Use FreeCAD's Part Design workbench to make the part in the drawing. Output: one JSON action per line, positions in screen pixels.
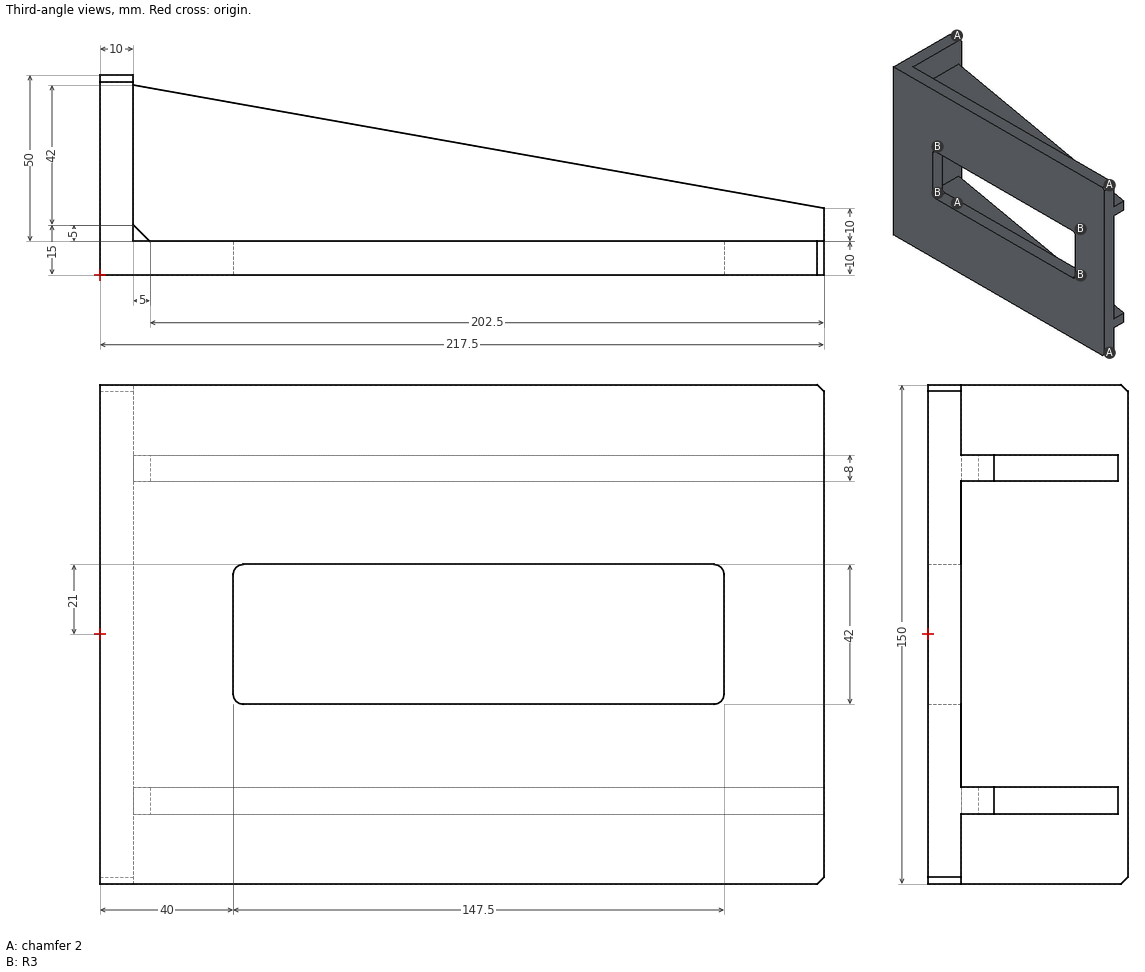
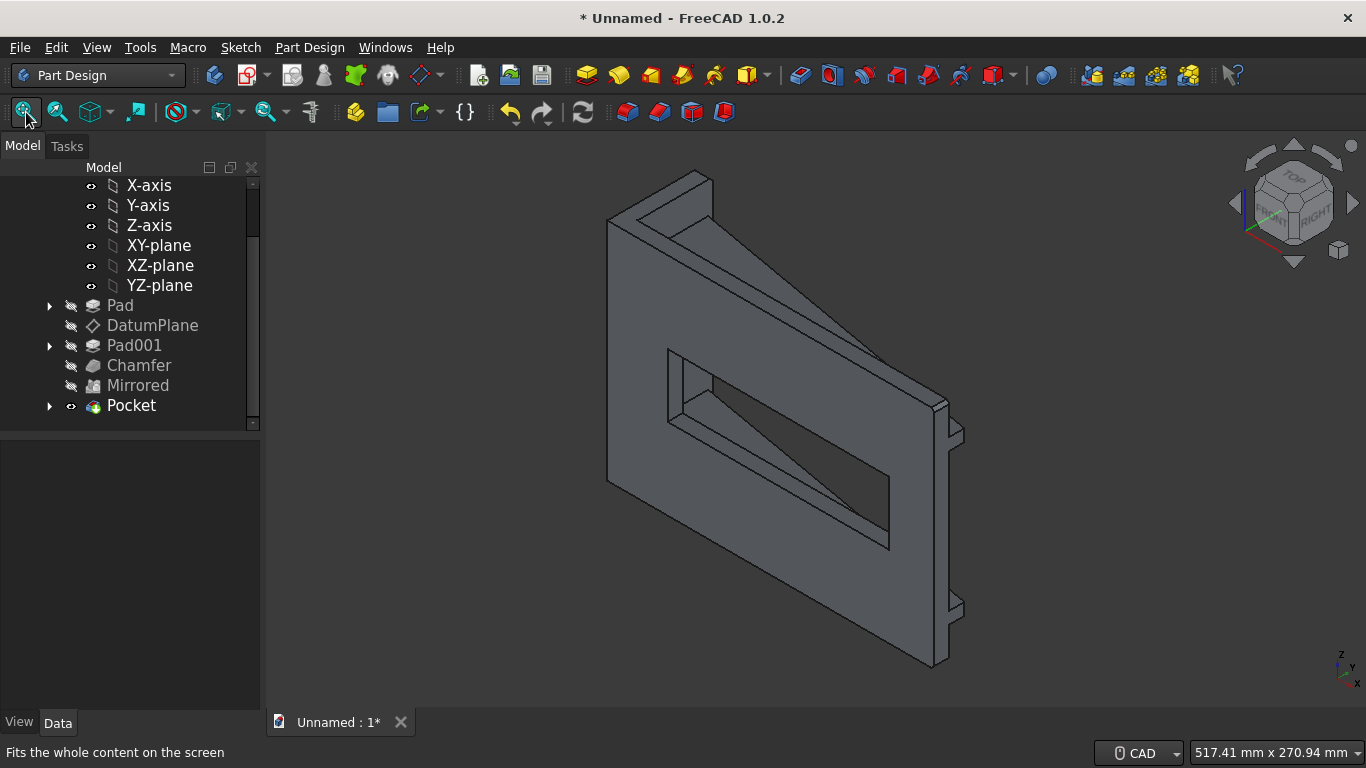
{"action": "key", "text": "2"}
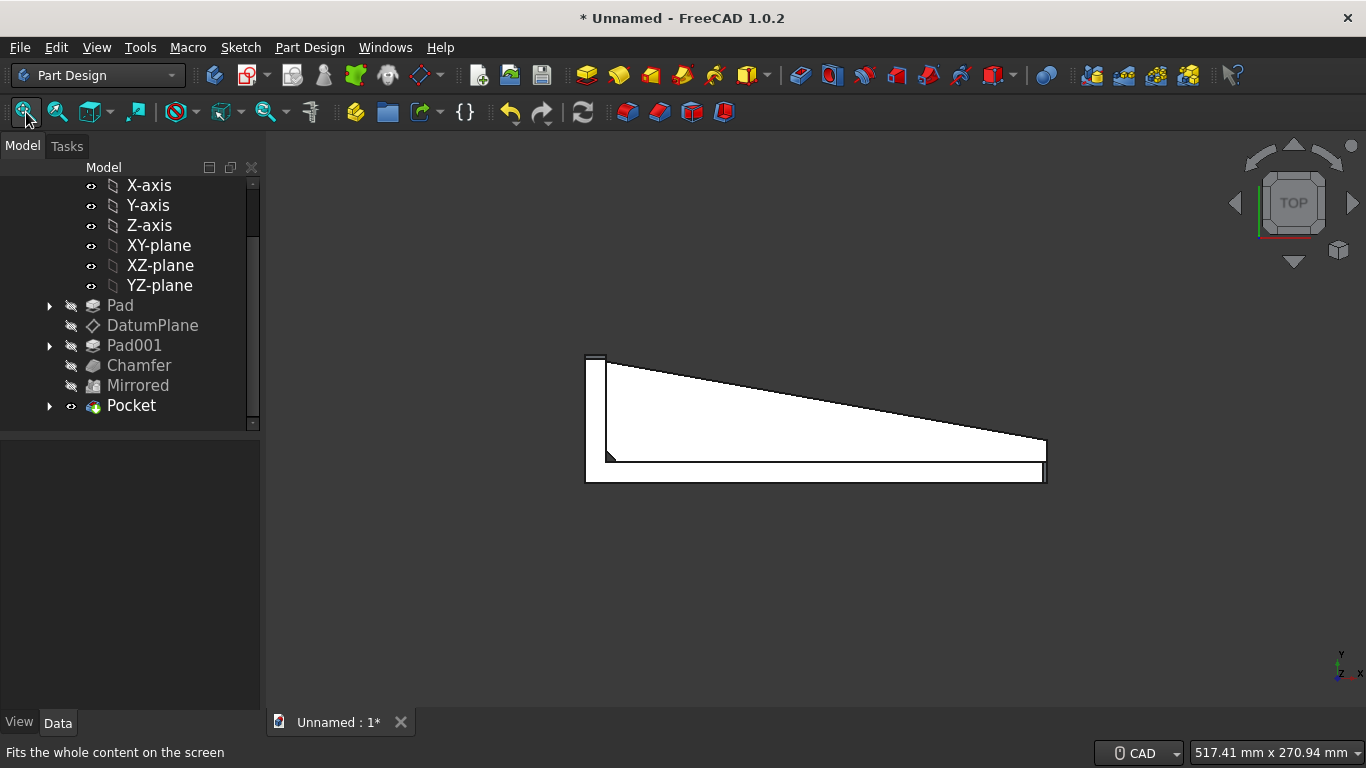
{"action": "left_click", "coordinate": [26, 112]}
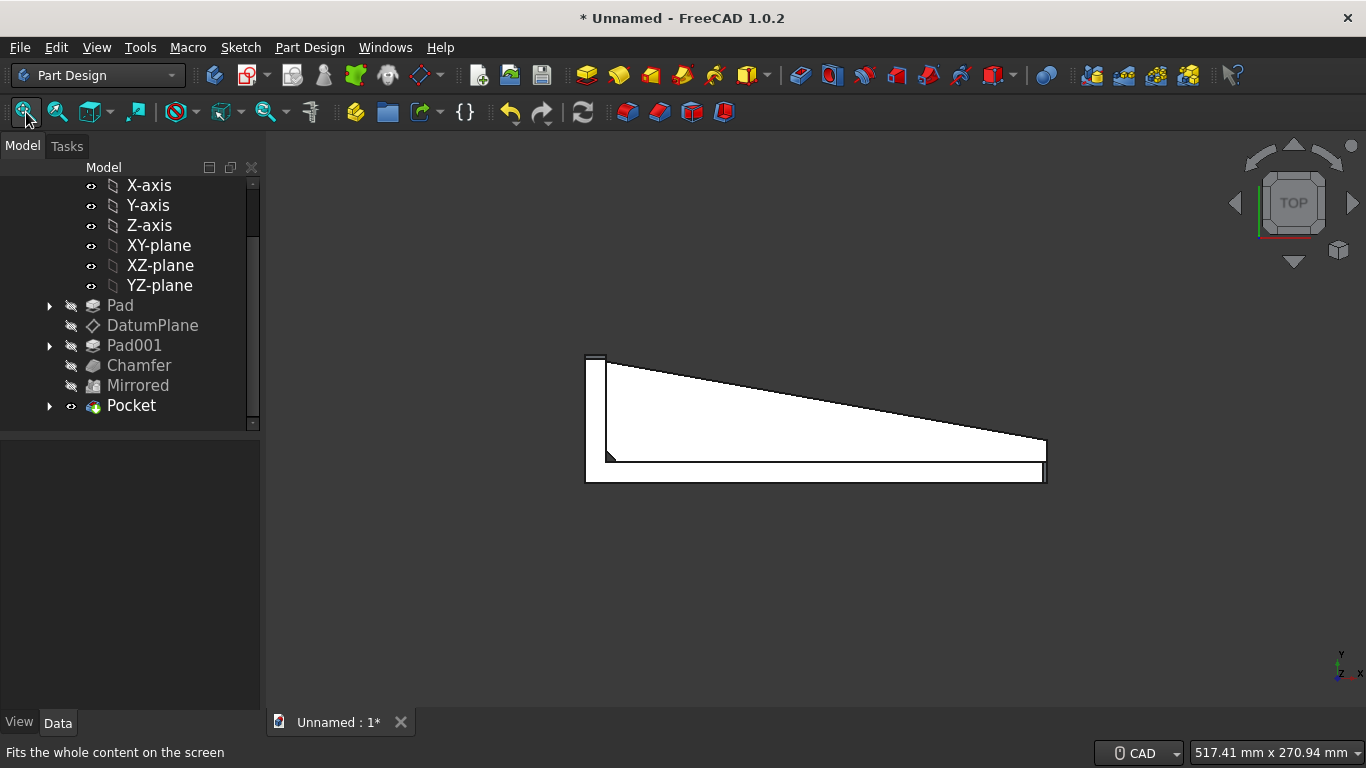
{"action": "scroll", "coordinate": [983, 471], "scroll_direction": "up", "scroll_amount": 4}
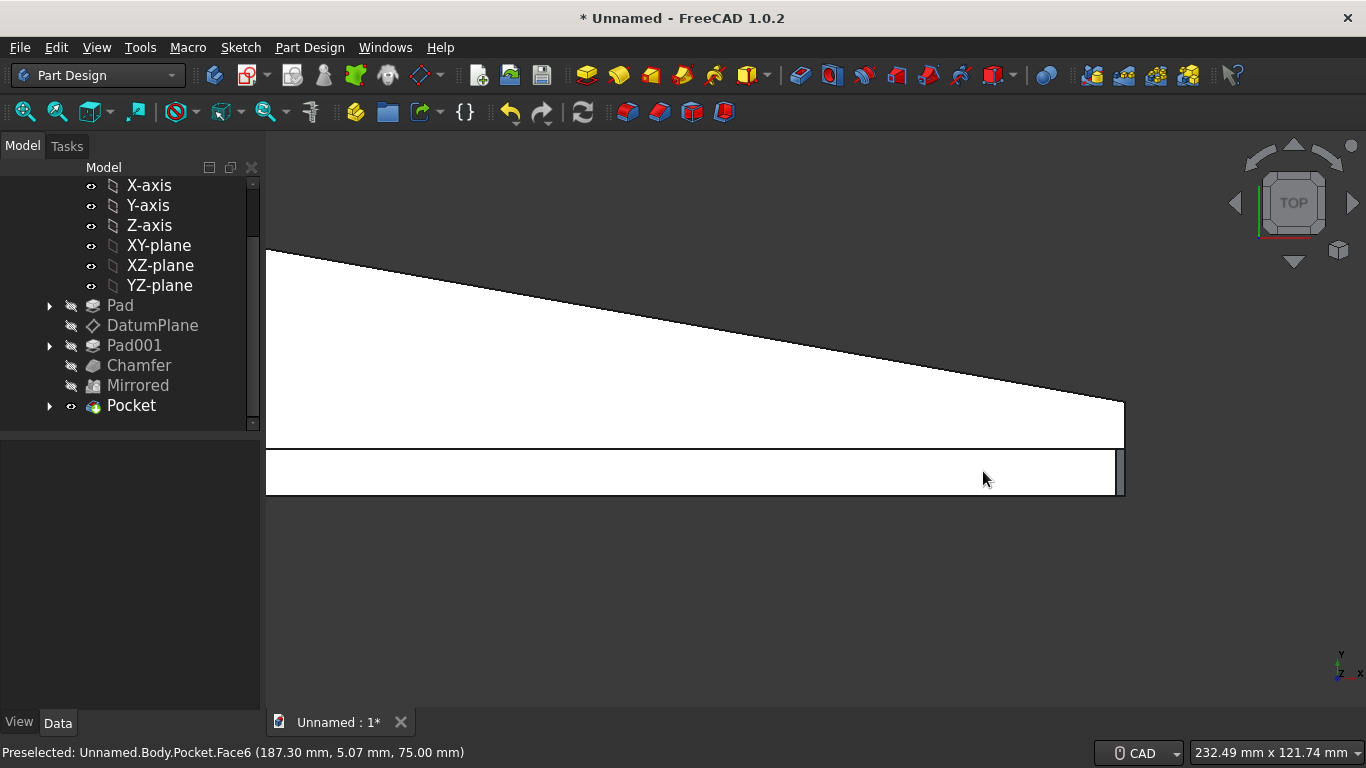
{"action": "left_click", "coordinate": [26, 112]}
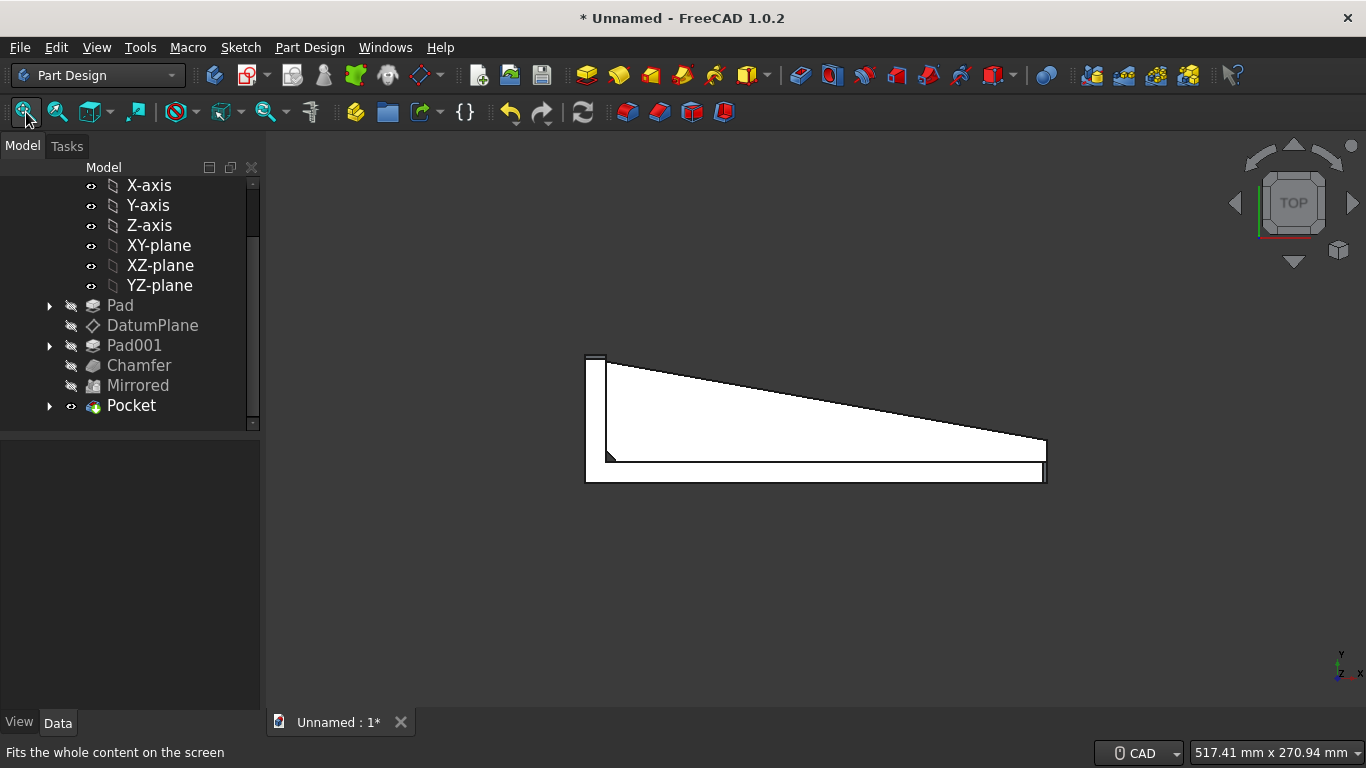
{"action": "key", "text": "1"}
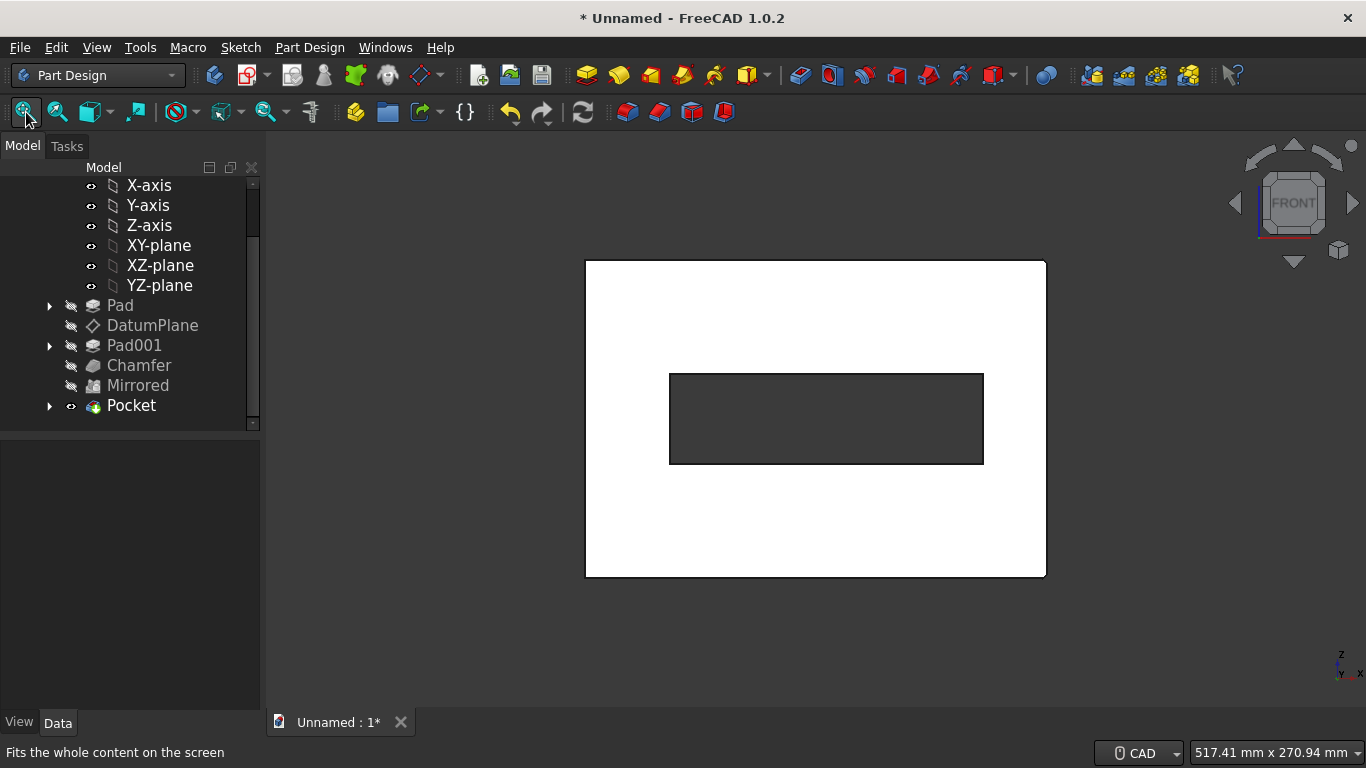
{"action": "scroll", "coordinate": [983, 463], "scroll_direction": "up", "scroll_amount": 4}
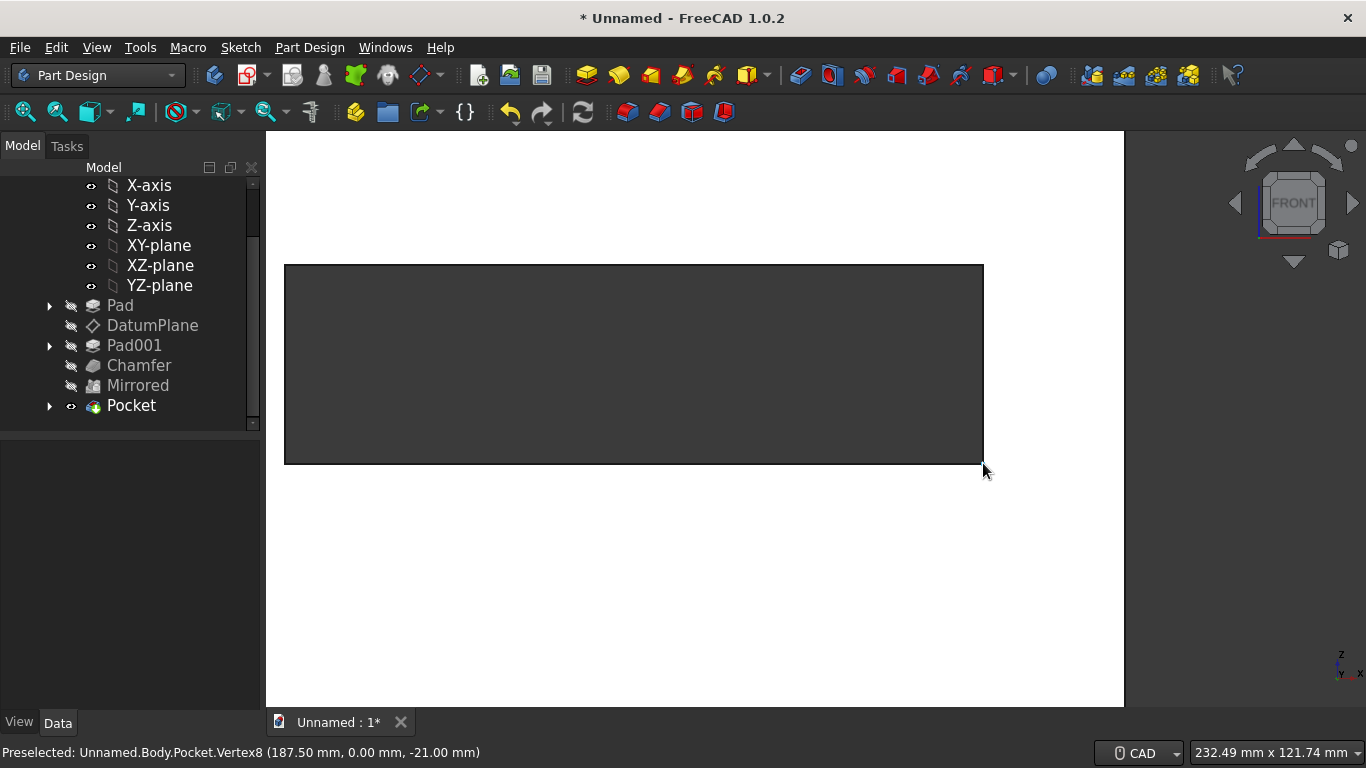
{"action": "left_click", "coordinate": [26, 112]}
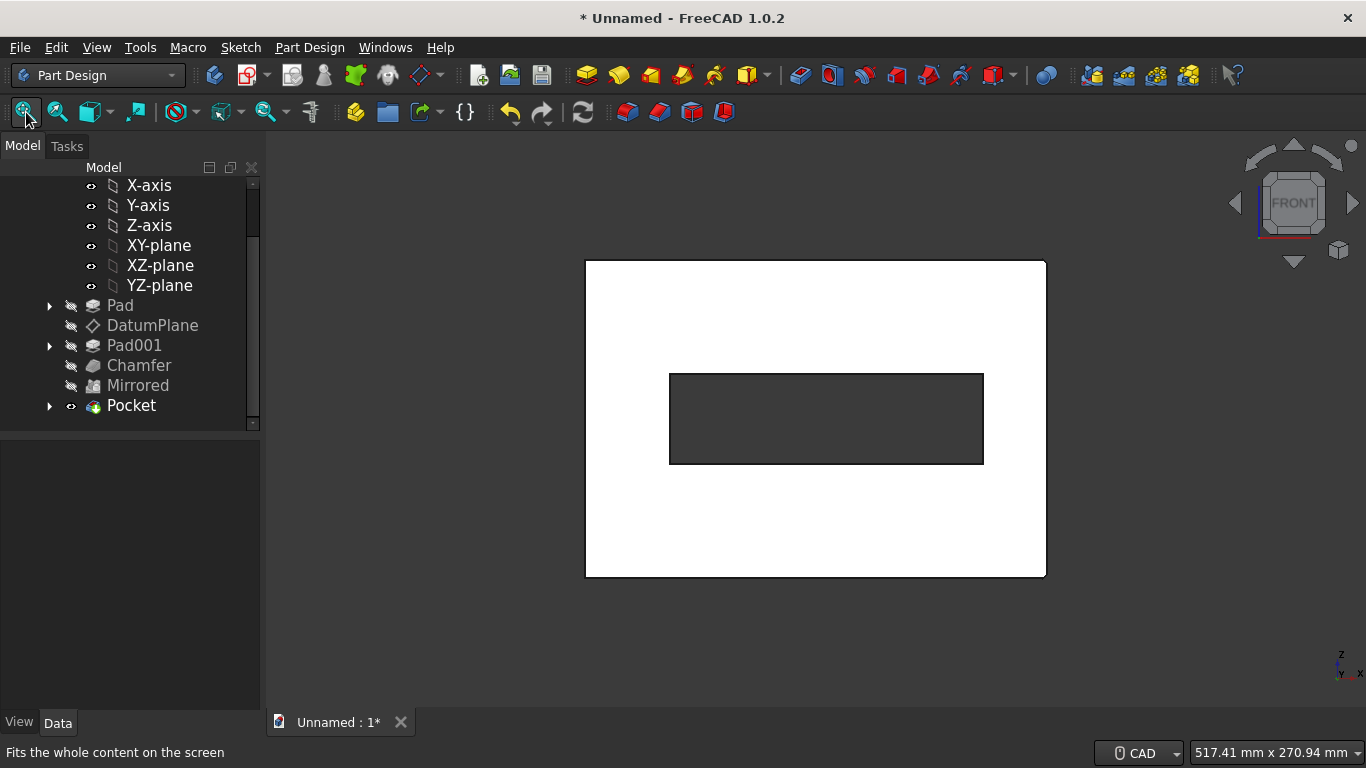
{"action": "key", "text": "3"}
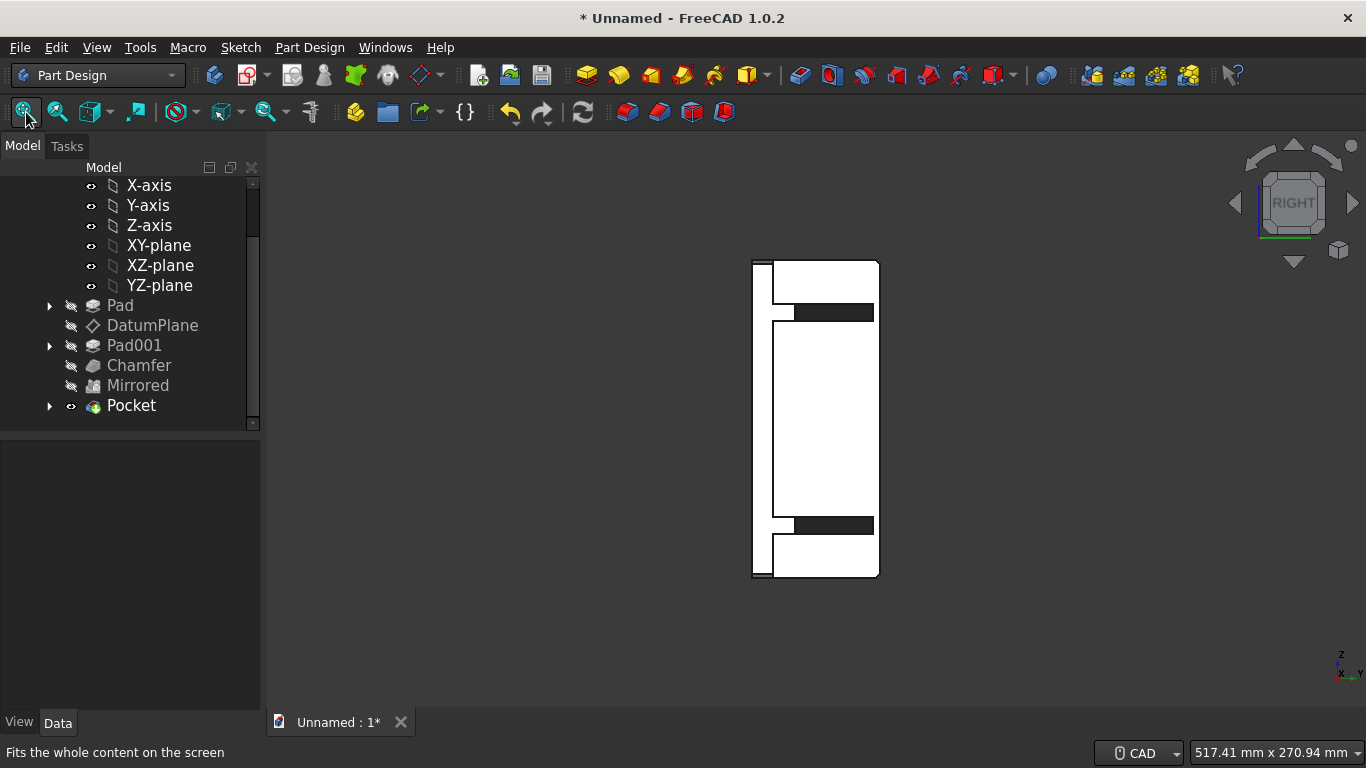
{"action": "scroll", "coordinate": [763, 463], "scroll_direction": "up", "scroll_amount": 4}